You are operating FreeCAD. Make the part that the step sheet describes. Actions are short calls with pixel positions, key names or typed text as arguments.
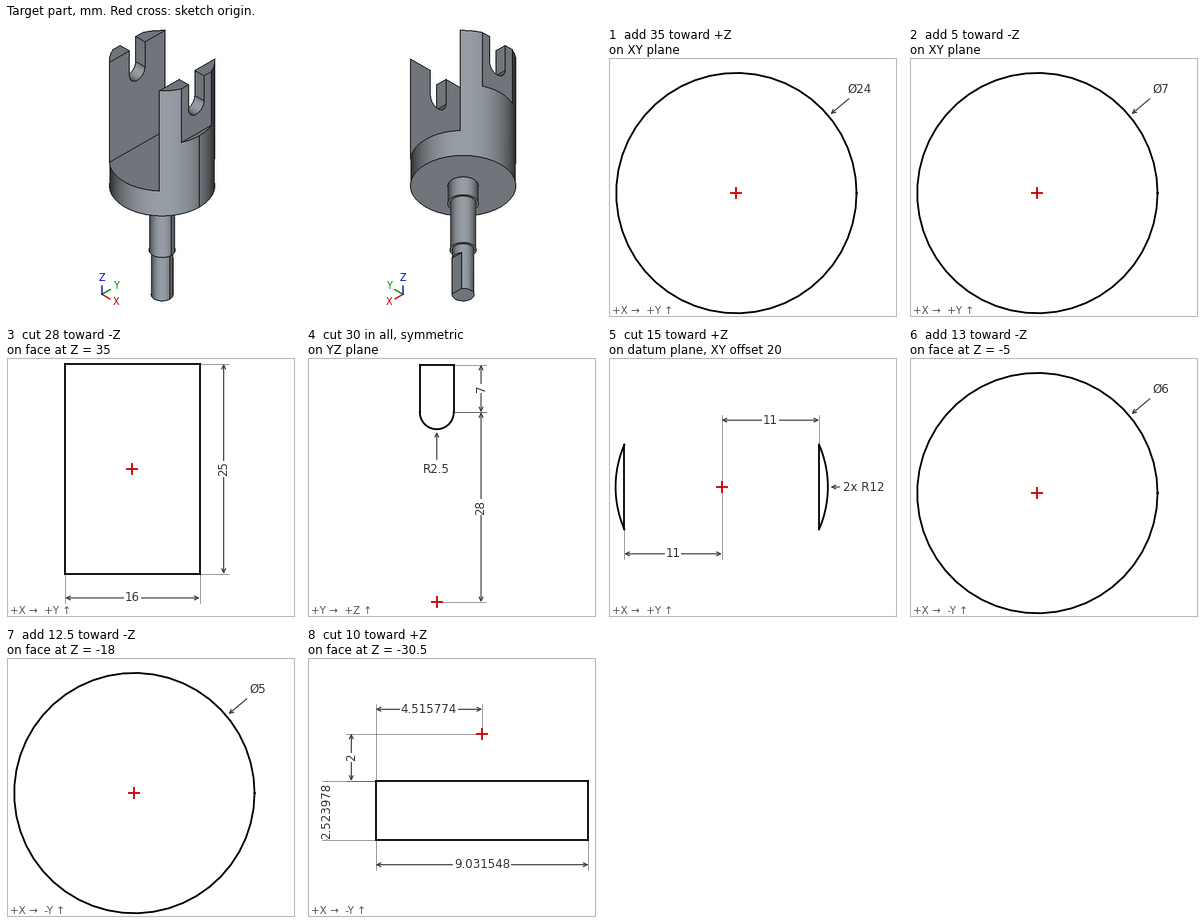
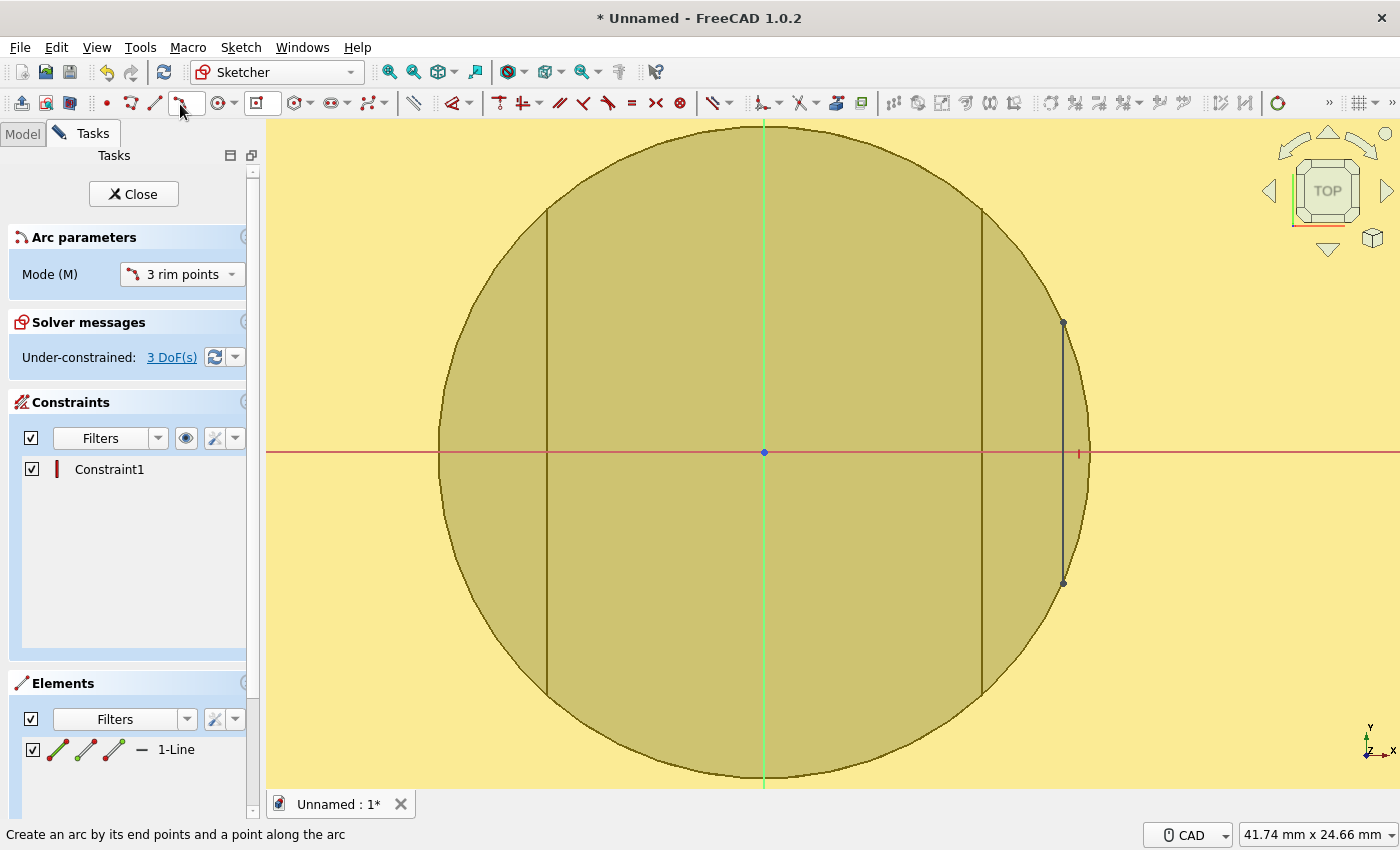
click(1063, 584)
click(1063, 323)
click(1089, 479)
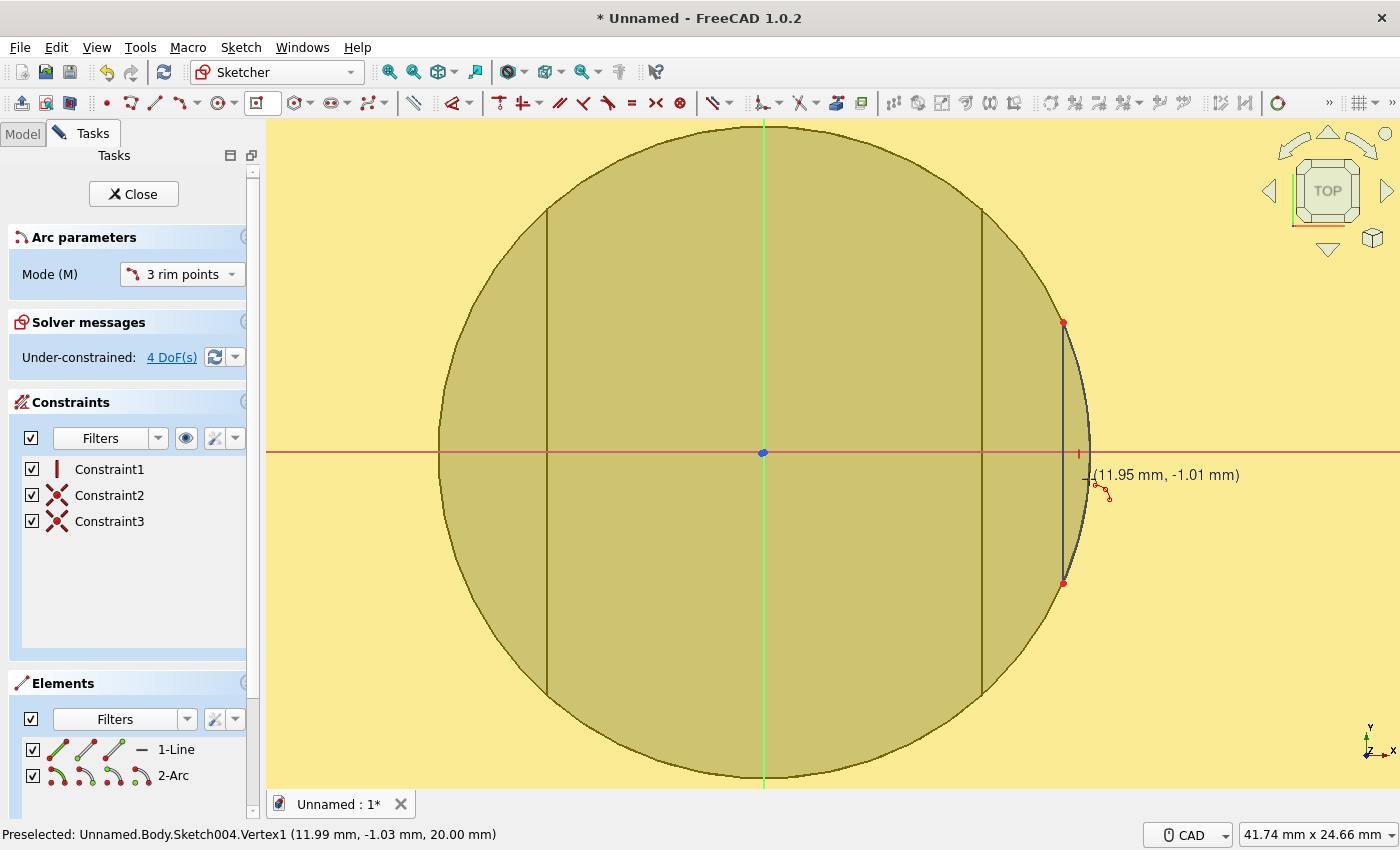
key(g)
key(l)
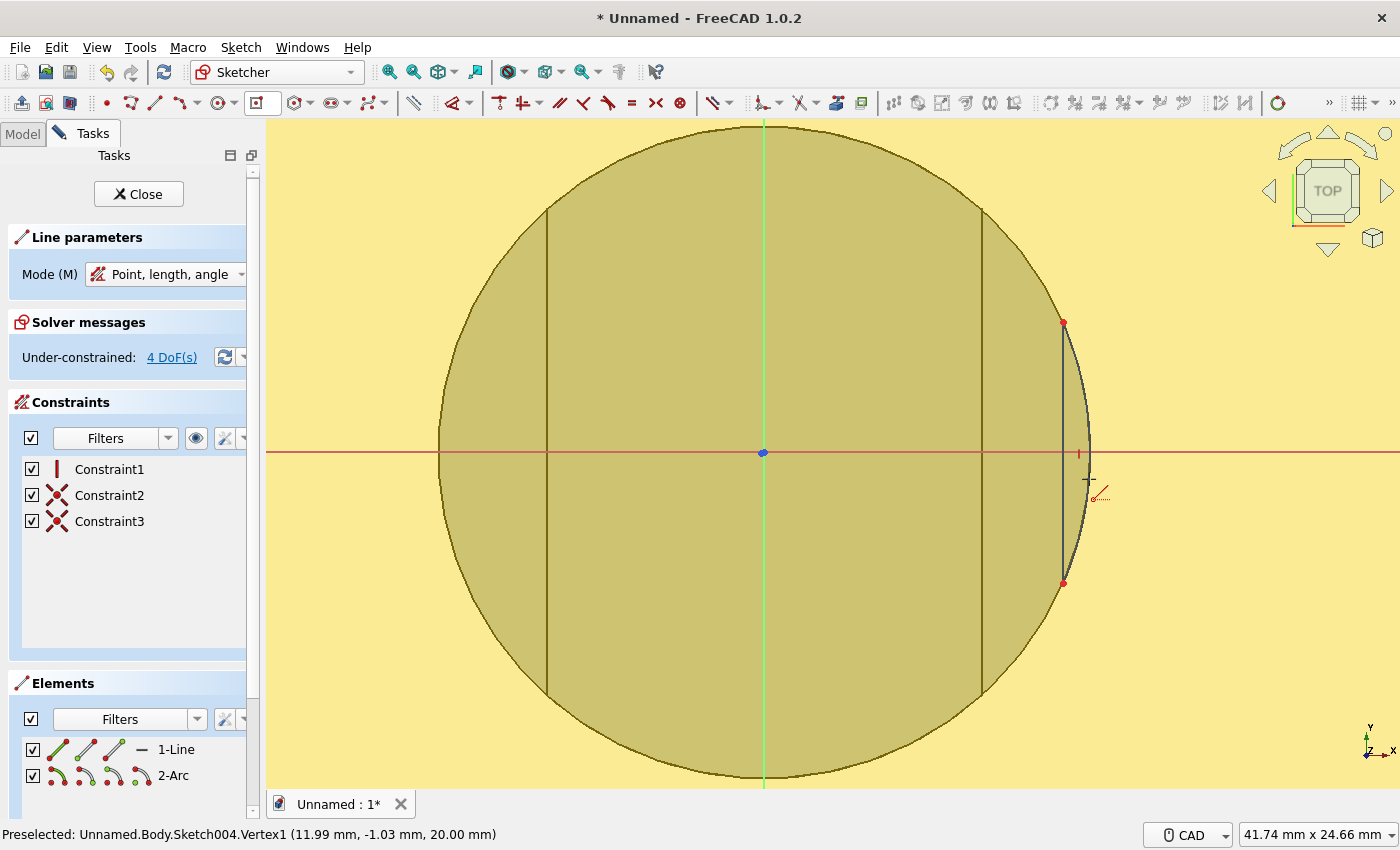
click(465, 583)
click(465, 322)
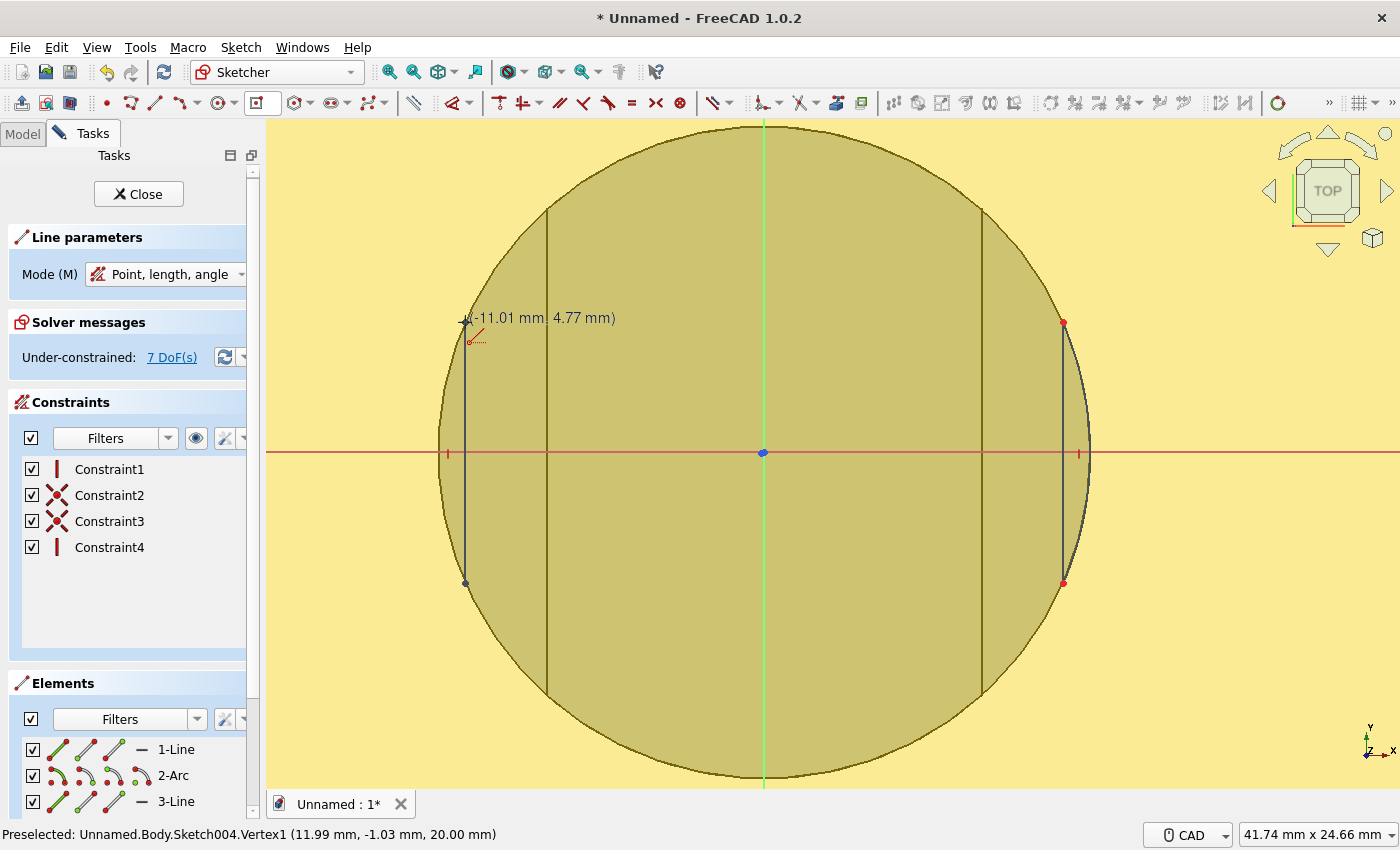
click(180, 104)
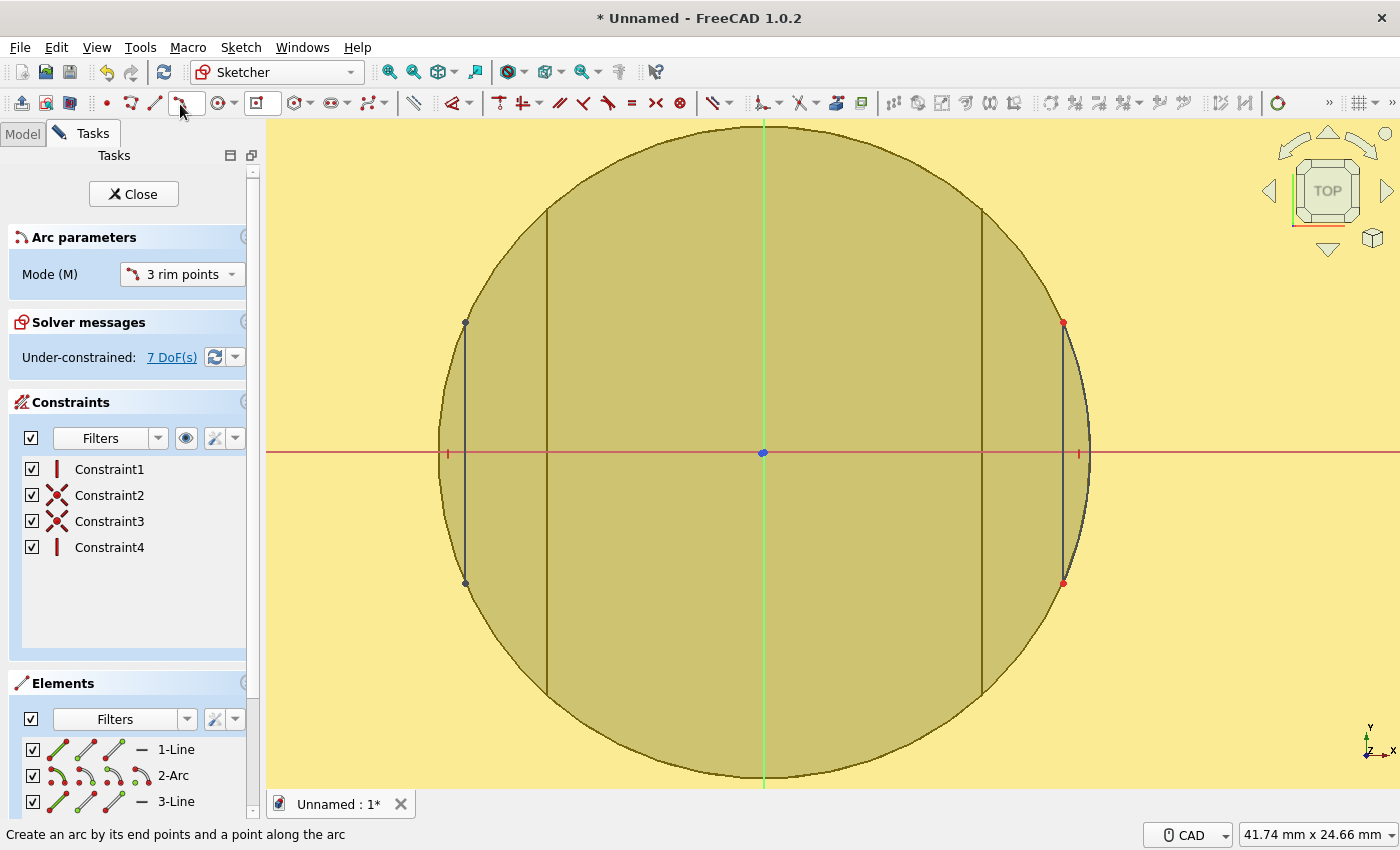
click(465, 323)
click(465, 584)
click(439, 426)
key(Escape)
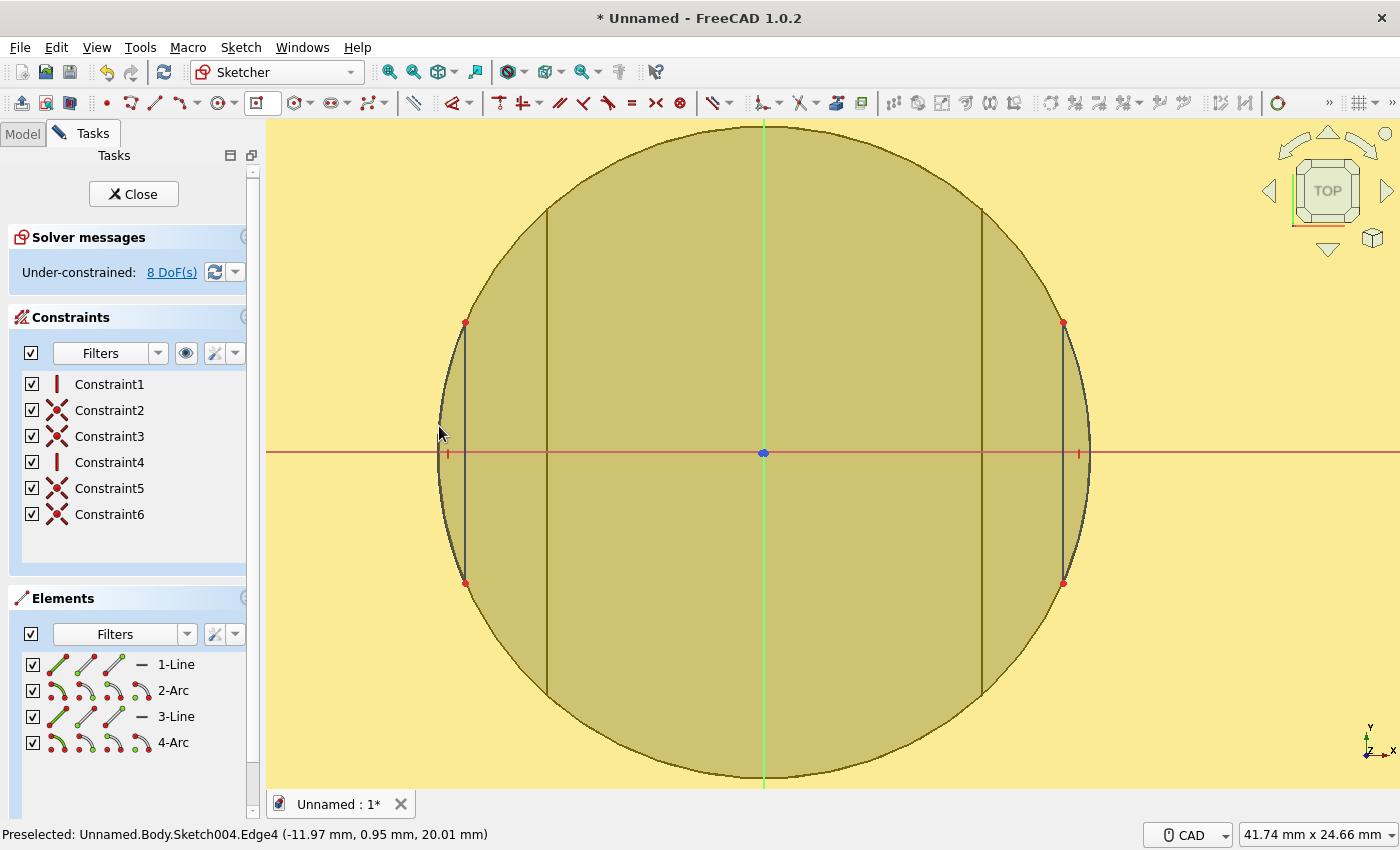
click(1086, 507)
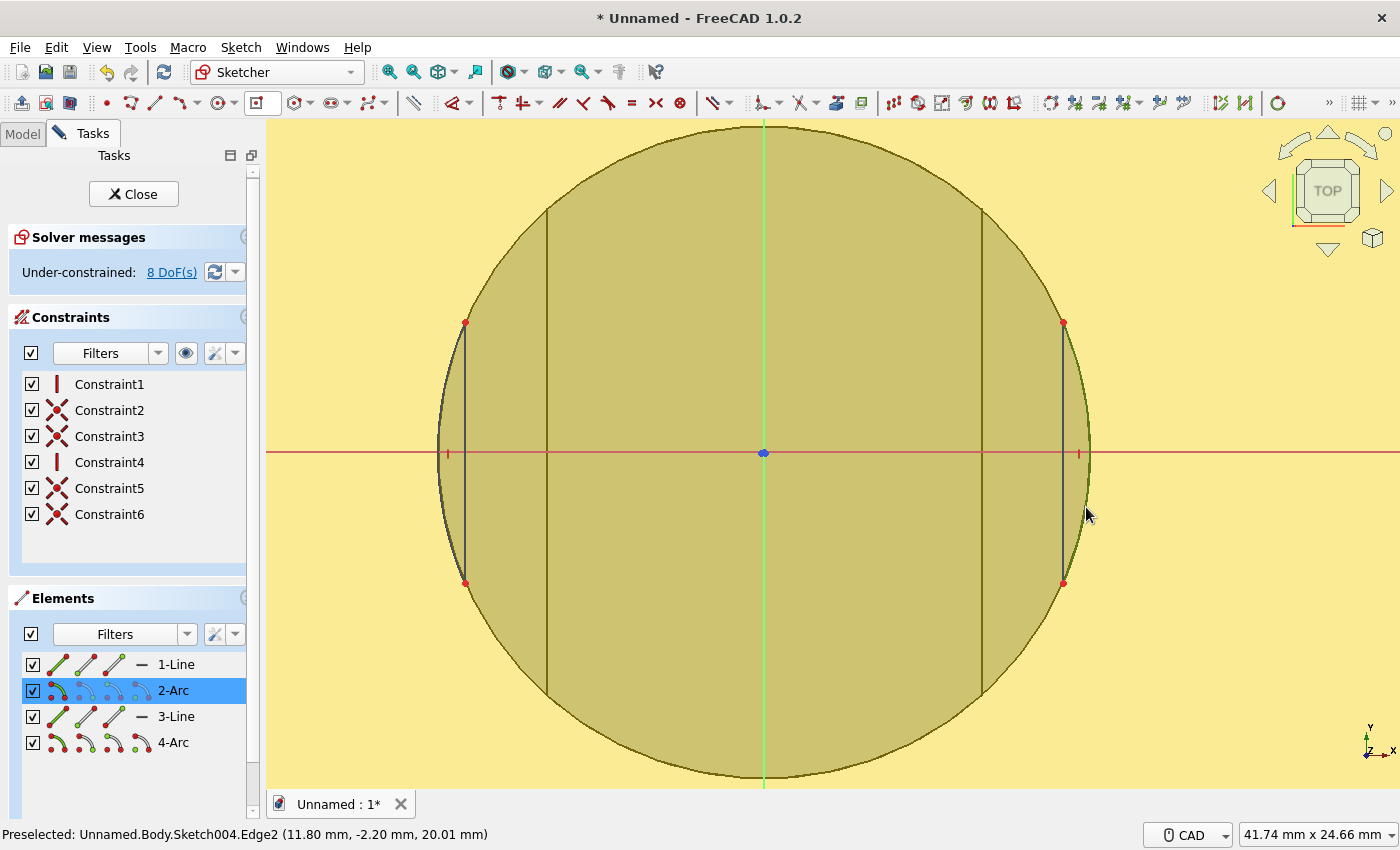
click(442, 400)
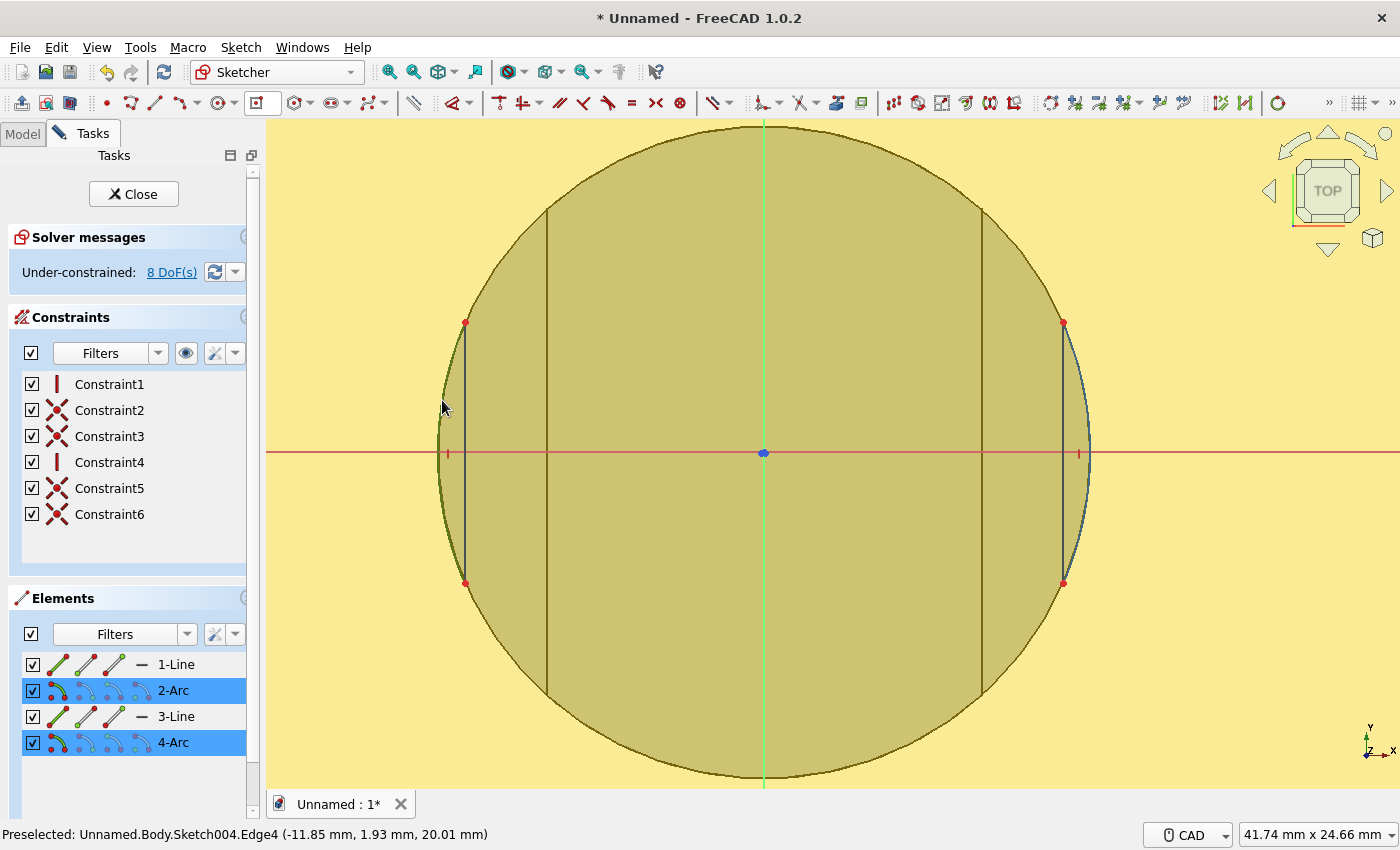
click(500, 104)